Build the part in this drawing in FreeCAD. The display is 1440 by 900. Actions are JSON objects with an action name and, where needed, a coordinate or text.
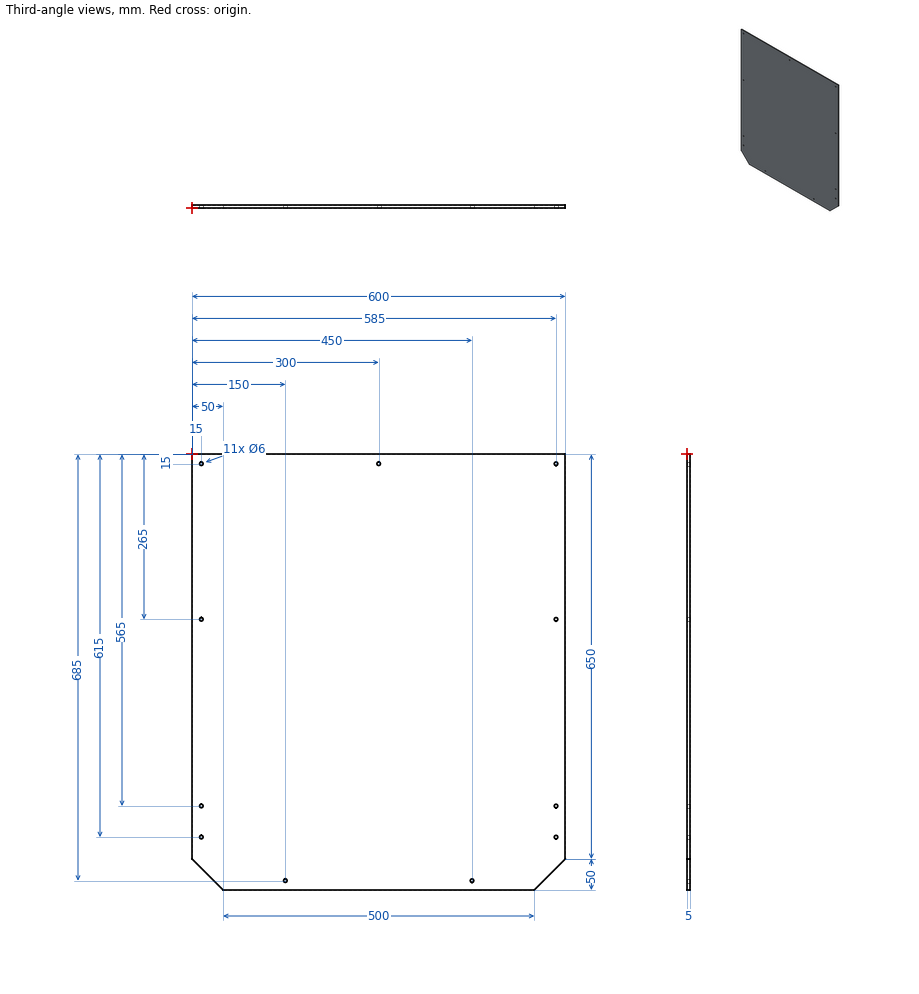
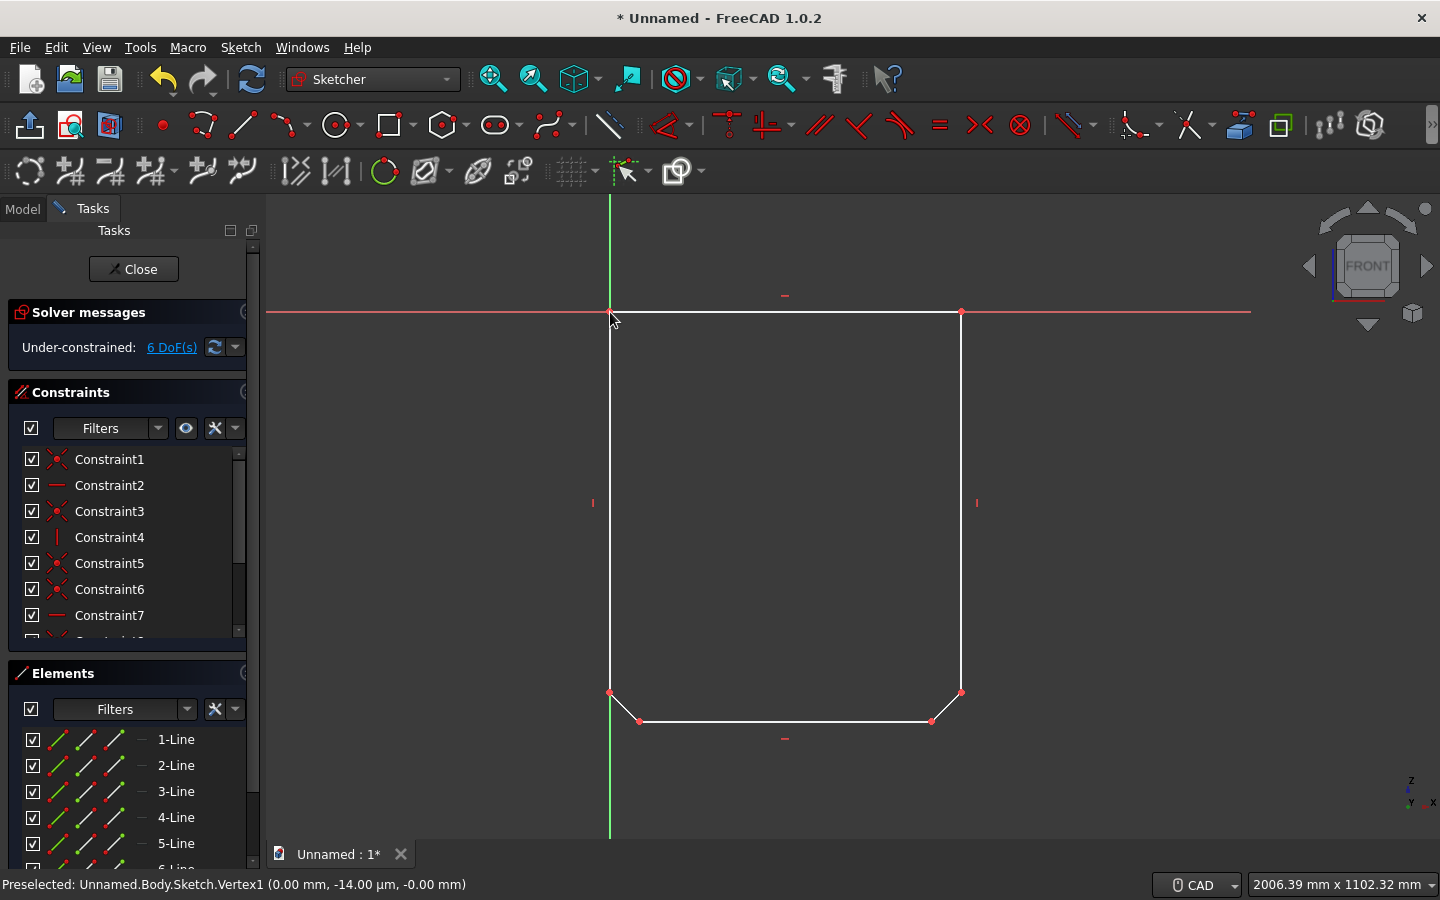
{"action": "left_click", "coordinate": [664, 126]}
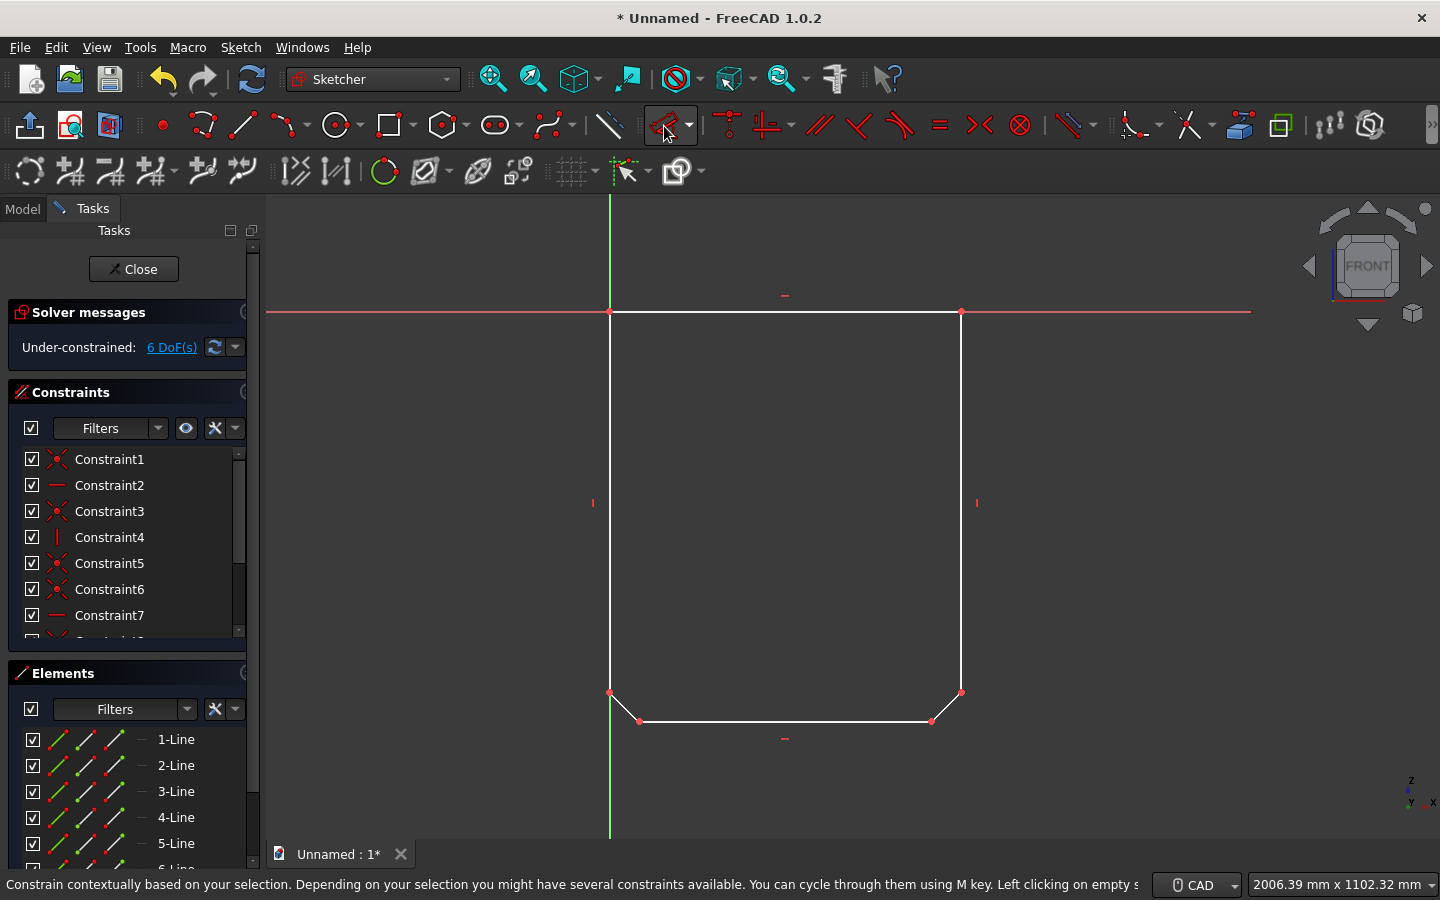
{"action": "left_click", "coordinate": [715, 312]}
{"action": "left_click", "coordinate": [785, 278]}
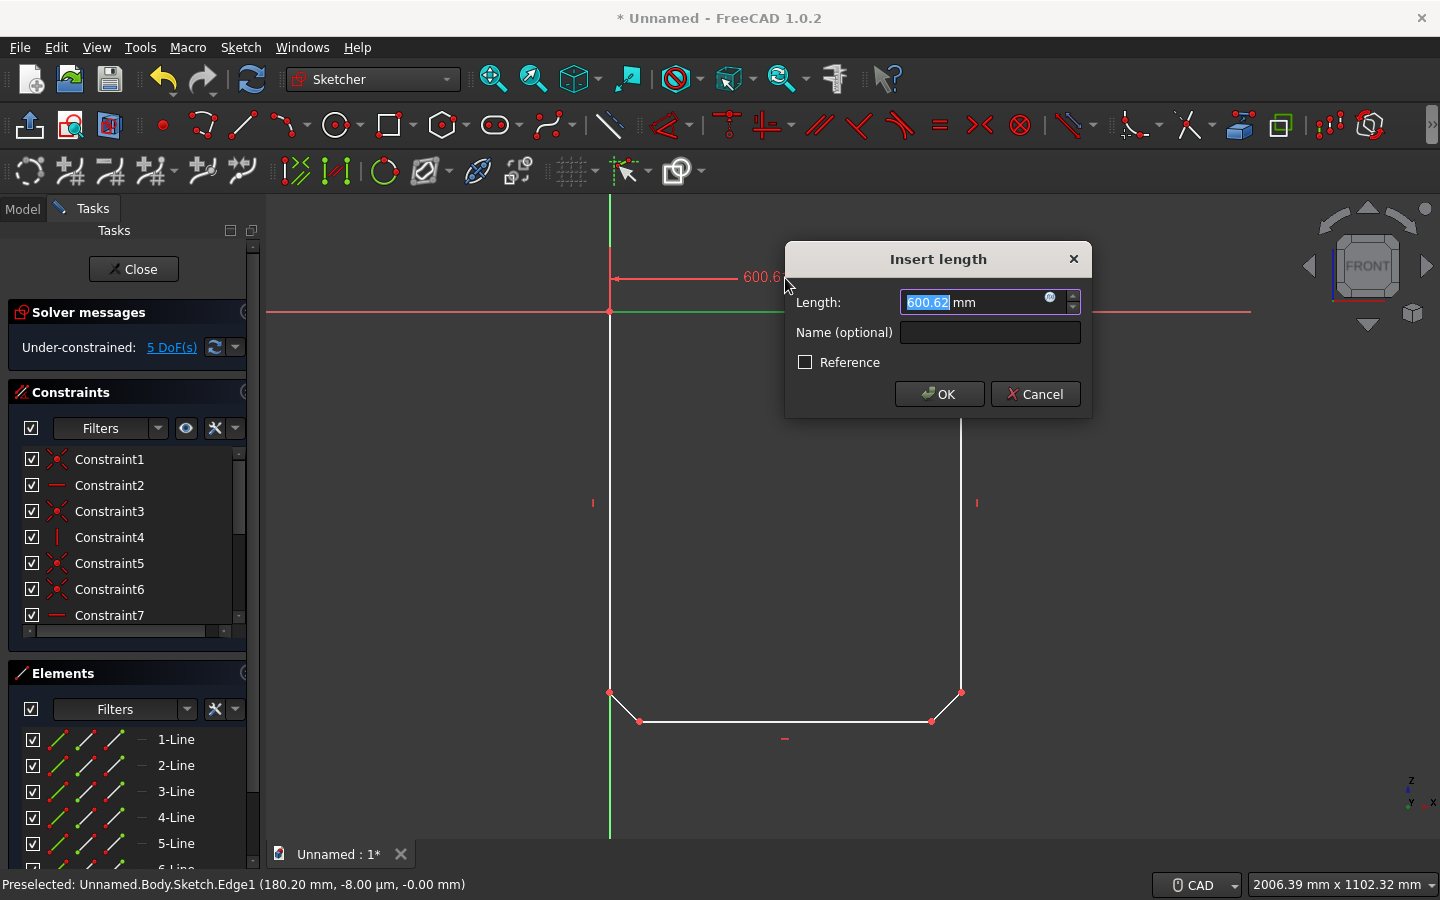
{"action": "type", "text": "600"}
{"action": "key", "text": "Return"}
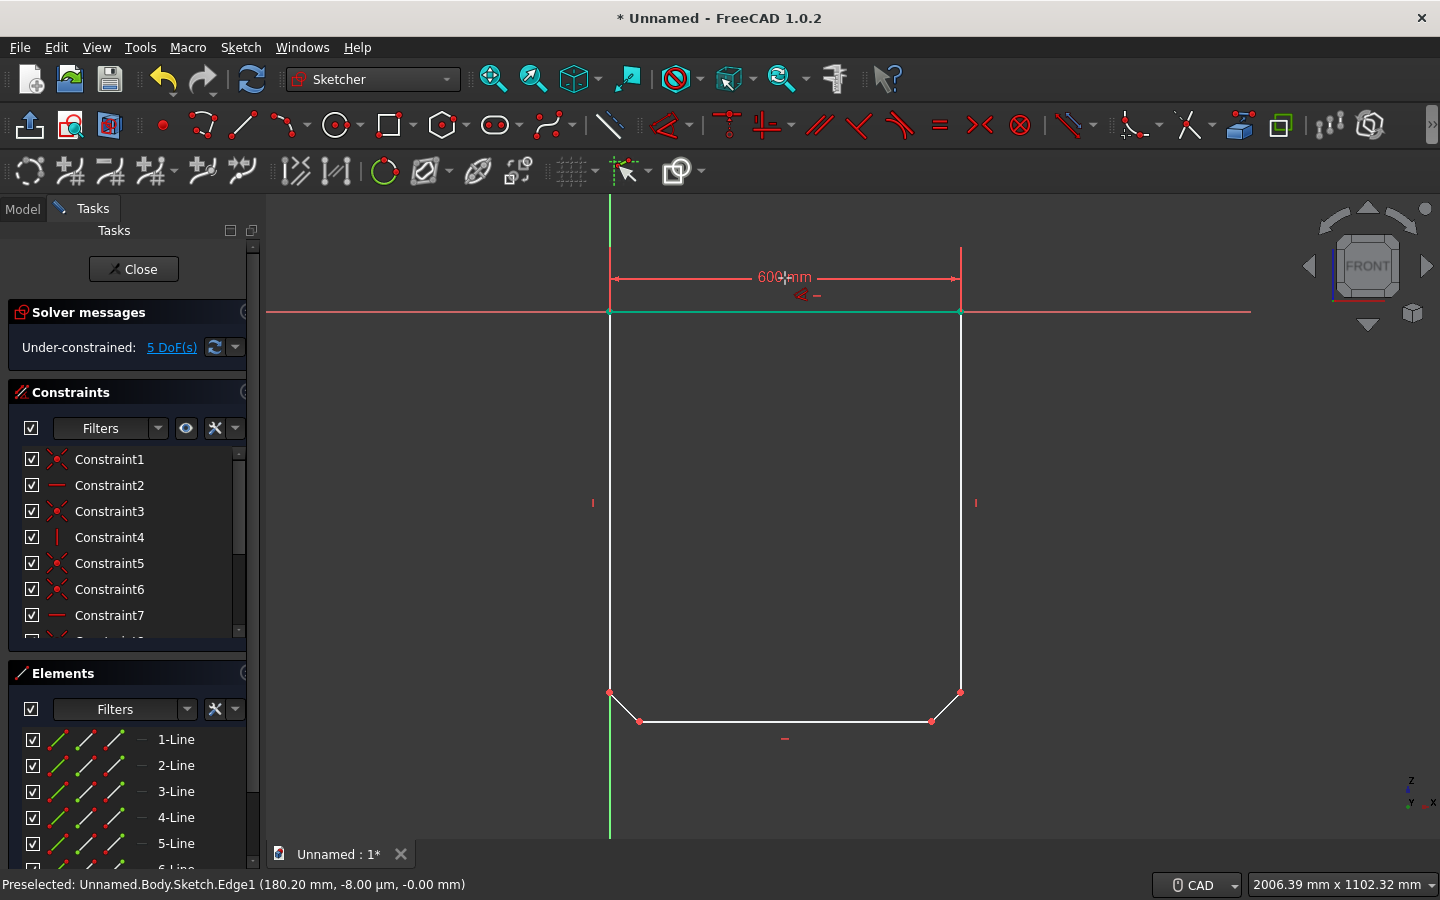
{"action": "left_click", "coordinate": [961, 426]}
{"action": "left_click", "coordinate": [995, 502]}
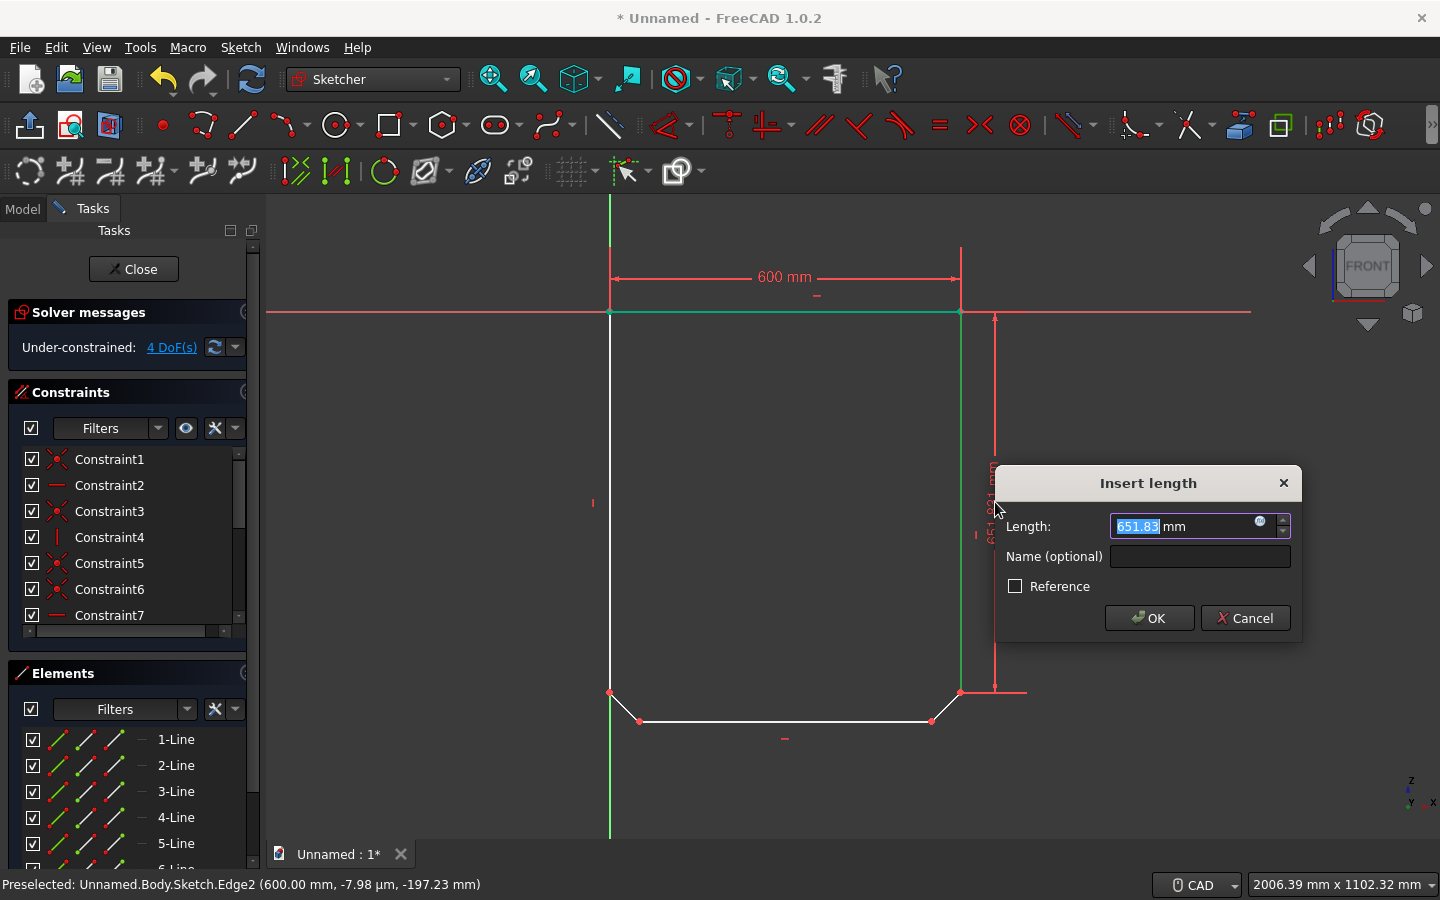
{"action": "type", "text": "650"}
{"action": "key", "text": "Return"}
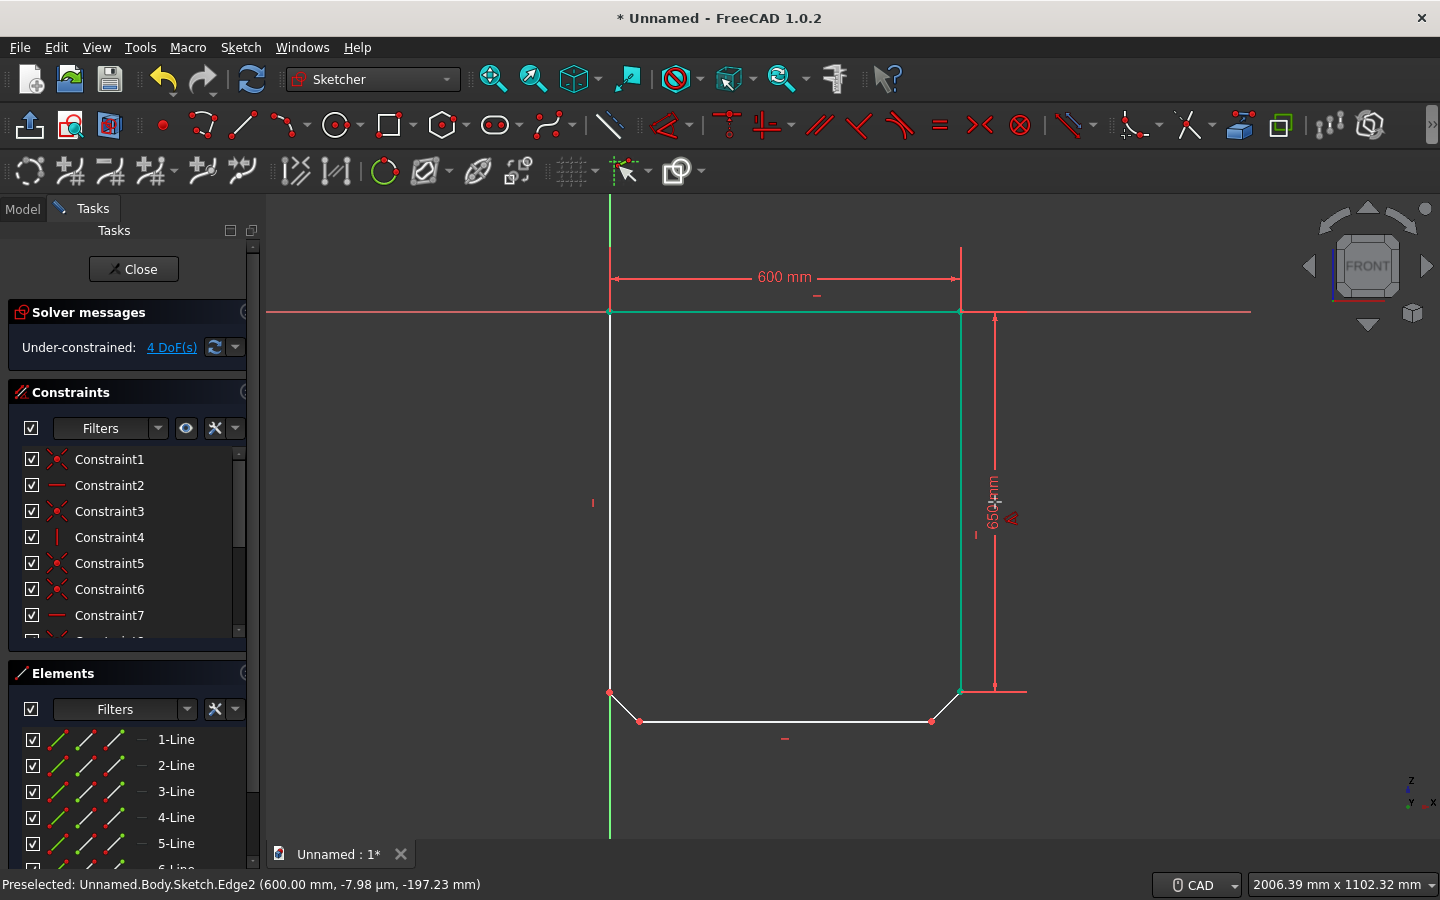
{"action": "left_click", "coordinate": [843, 722]}
{"action": "left_click", "coordinate": [785, 756]}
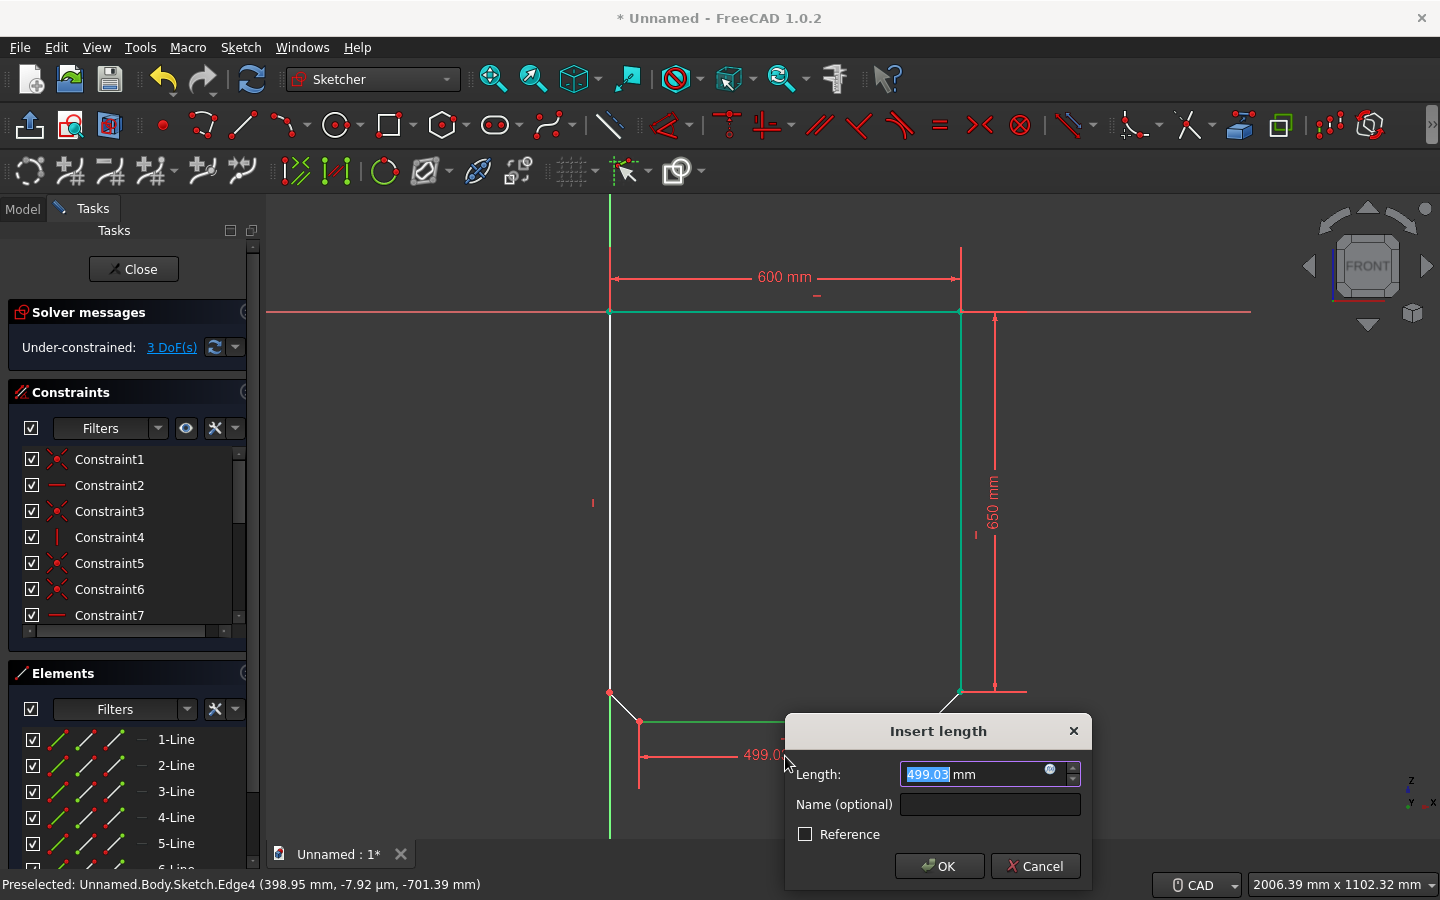
{"action": "type", "text": "500"}
{"action": "key", "text": "Return"}